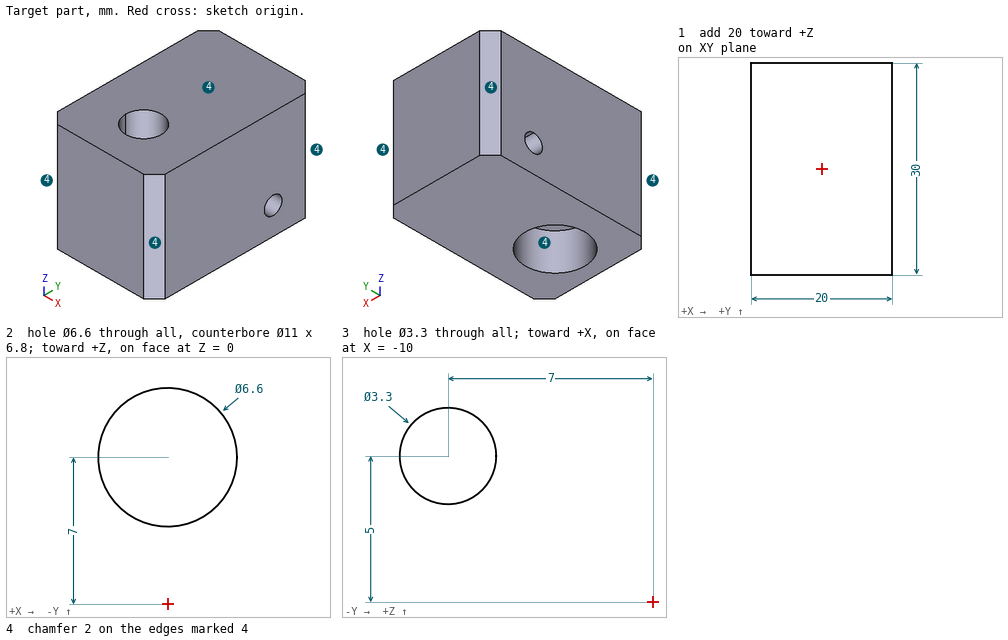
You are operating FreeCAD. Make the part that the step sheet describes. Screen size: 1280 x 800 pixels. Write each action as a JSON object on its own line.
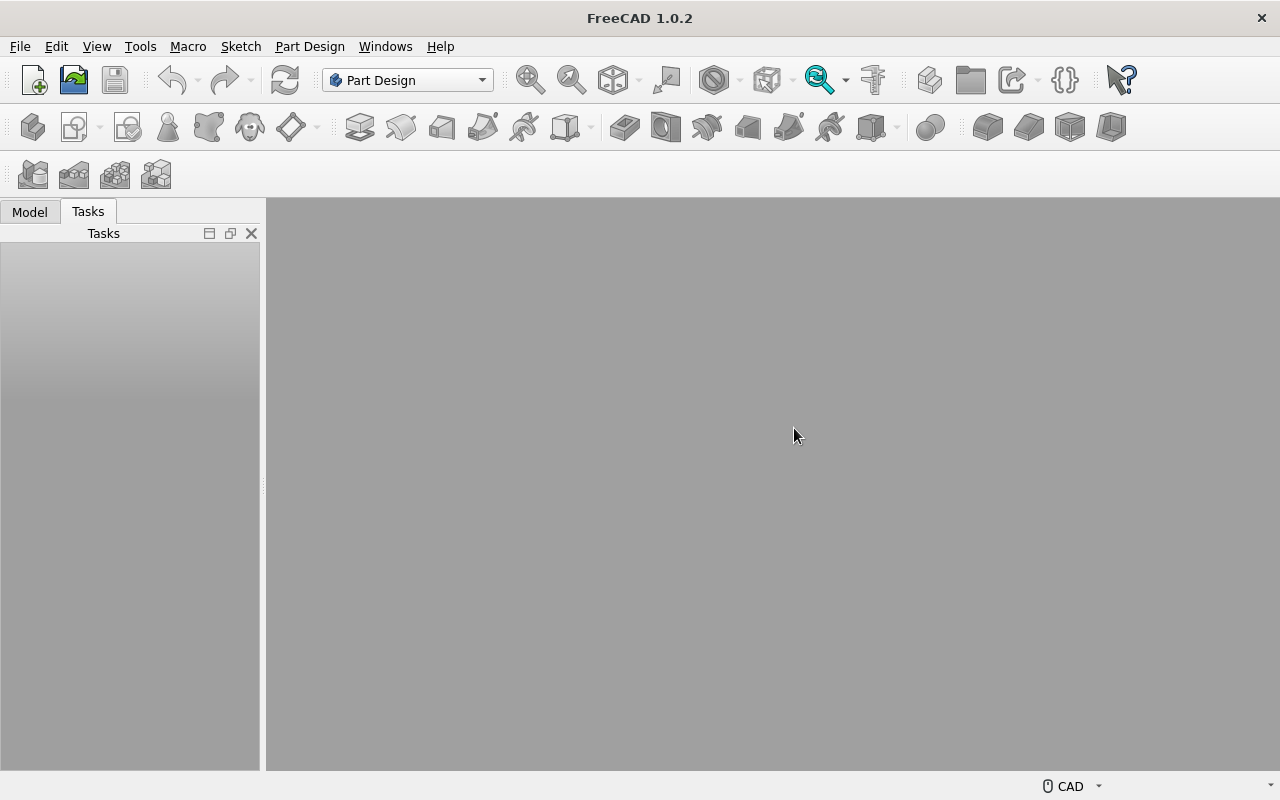
{"action": "key", "text": "ctrl+n"}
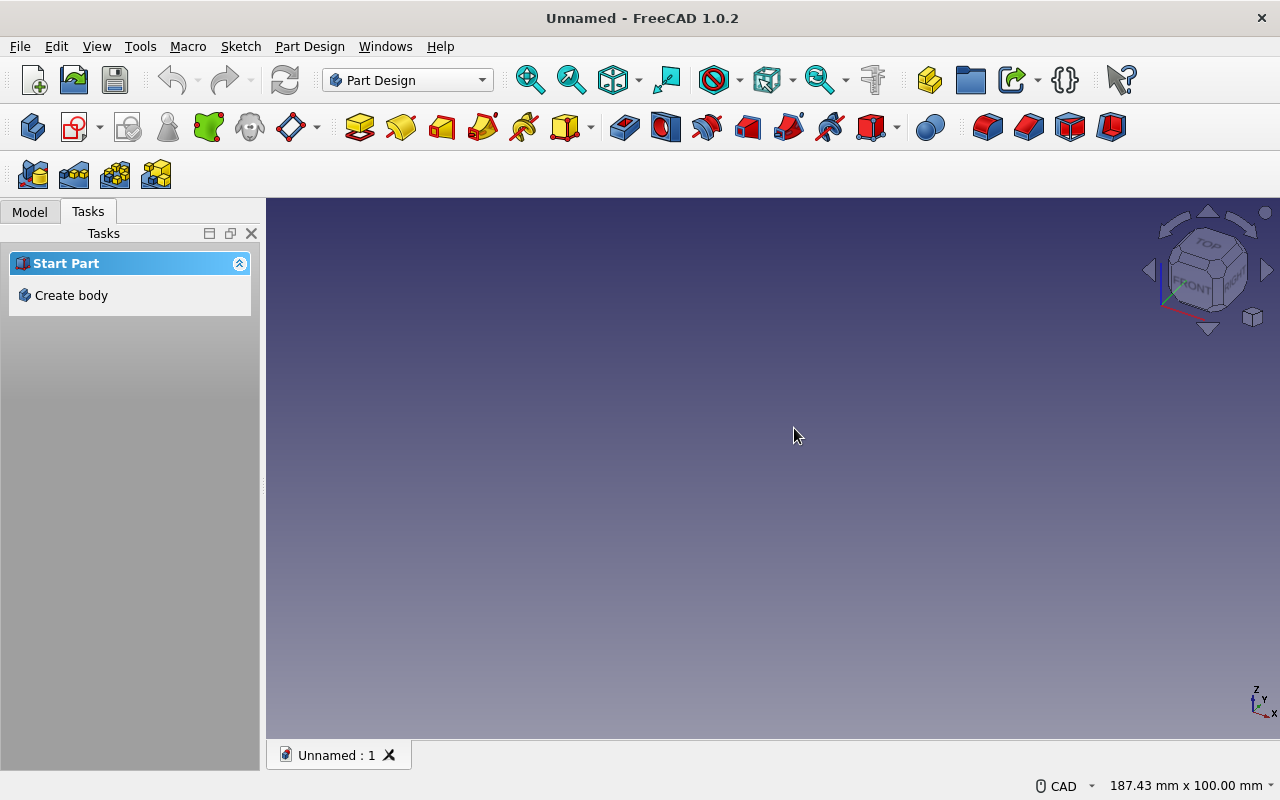
{"action": "left_click", "coordinate": [74, 128]}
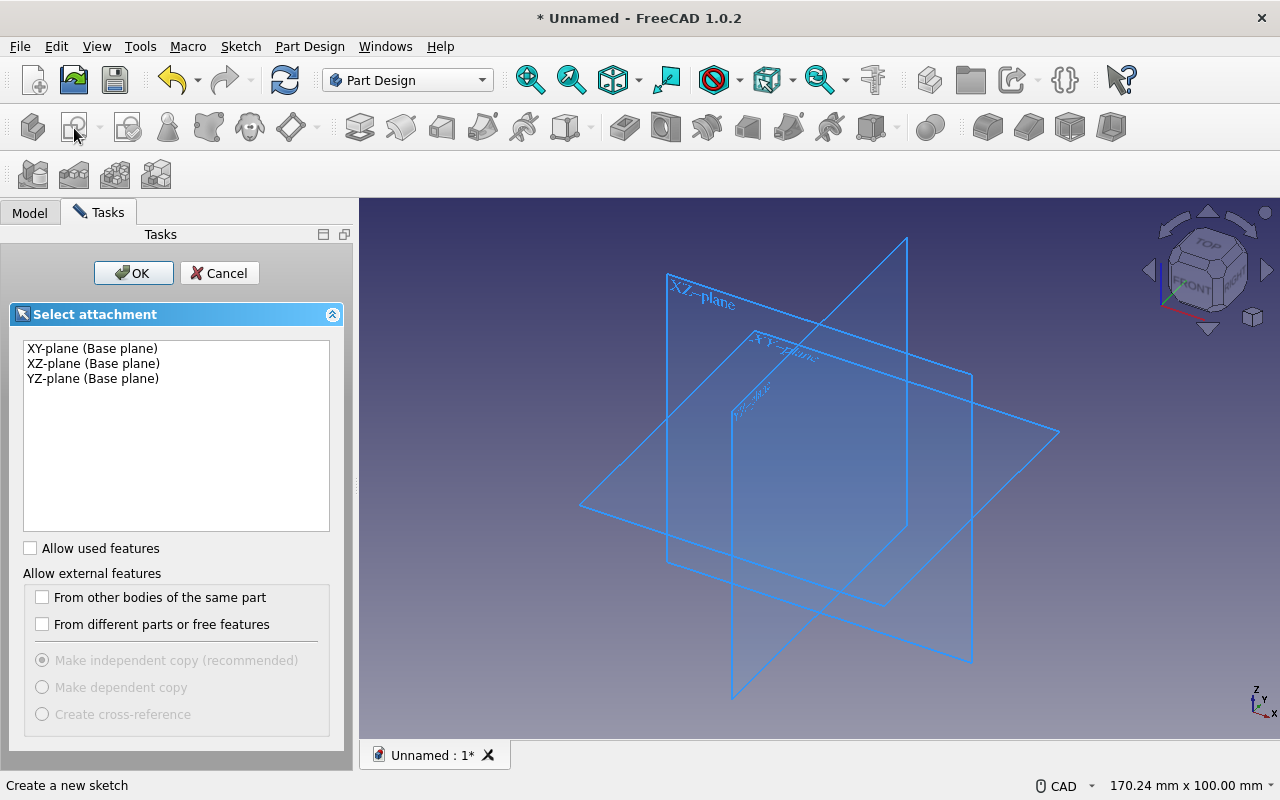
{"action": "left_click", "coordinate": [84, 348]}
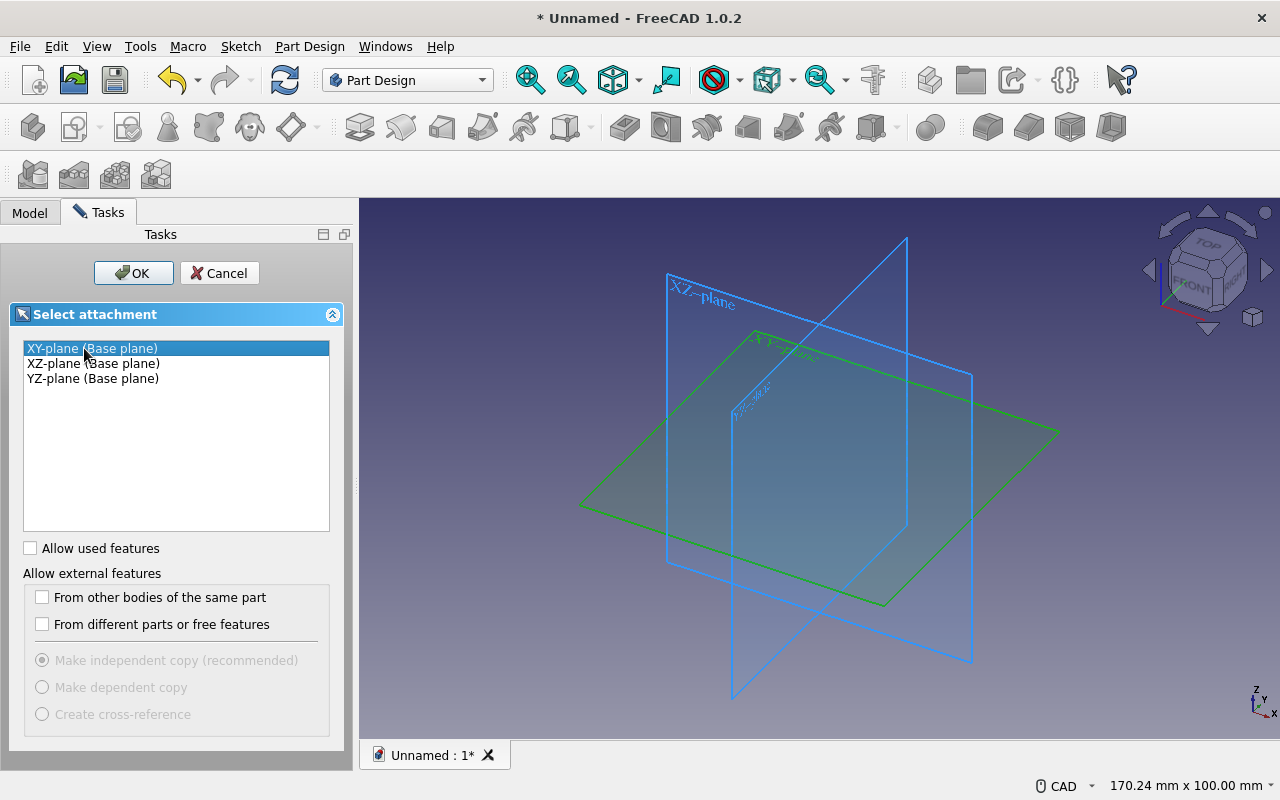
{"action": "left_click", "coordinate": [134, 273]}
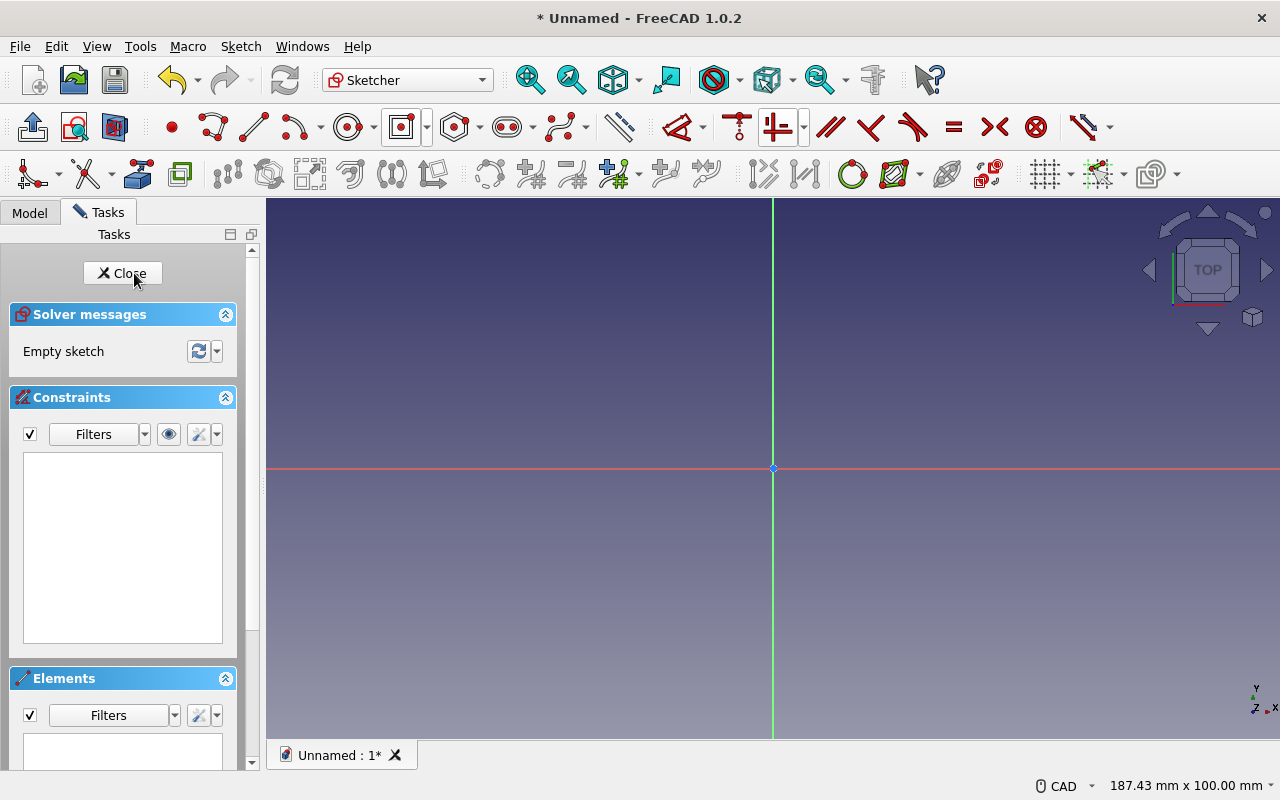
{"action": "scroll", "coordinate": [829, 469], "scroll_direction": "up", "scroll_amount": 4}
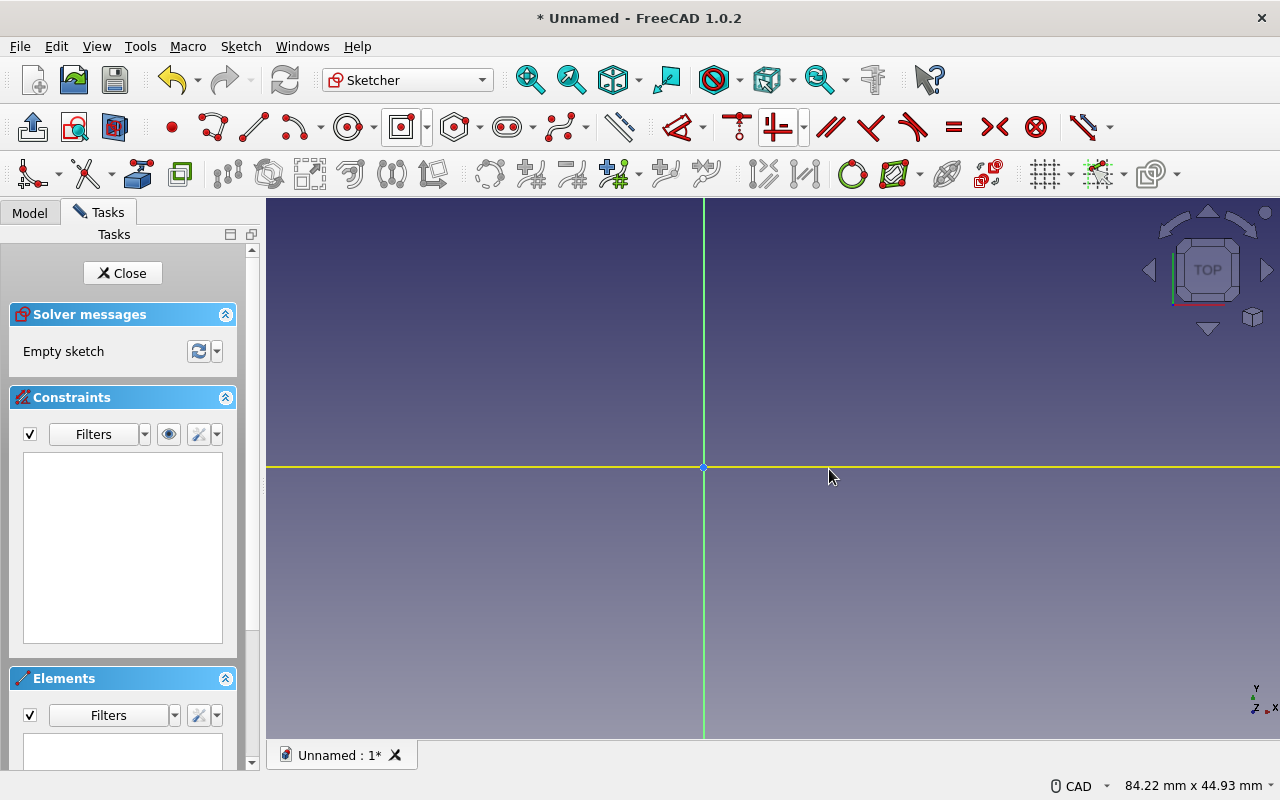
{"action": "key", "text": "g v"}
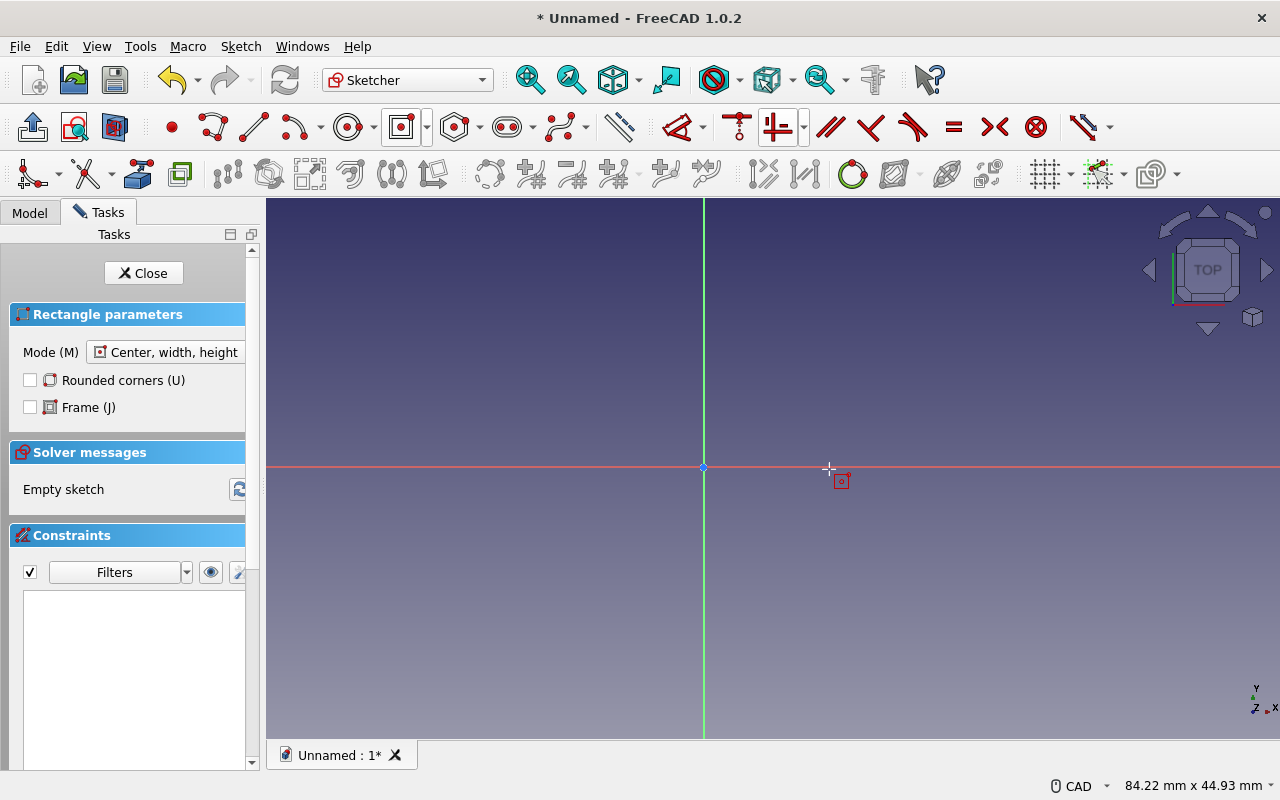
{"action": "left_click", "coordinate": [704, 467]}
{"action": "left_click", "coordinate": [824, 287]}
{"action": "key", "text": "Escape"}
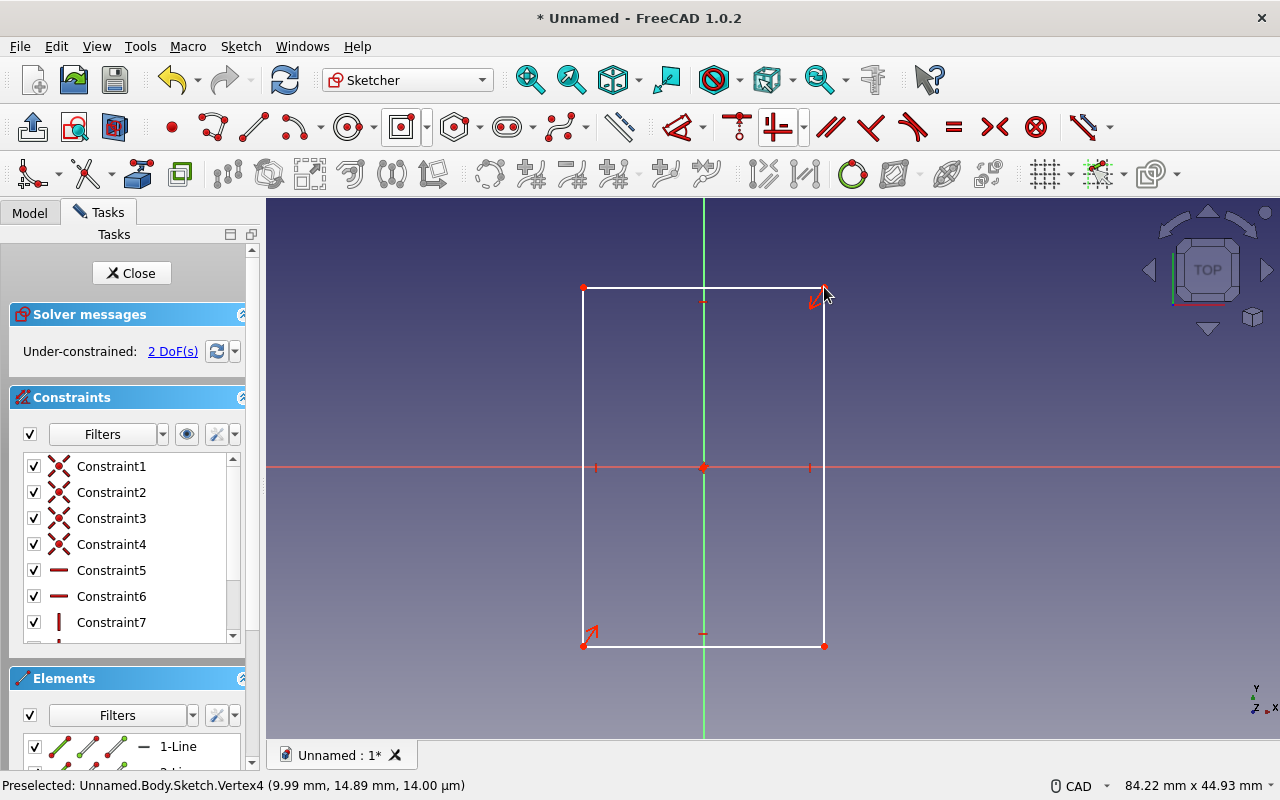
{"action": "left_click", "coordinate": [656, 647]}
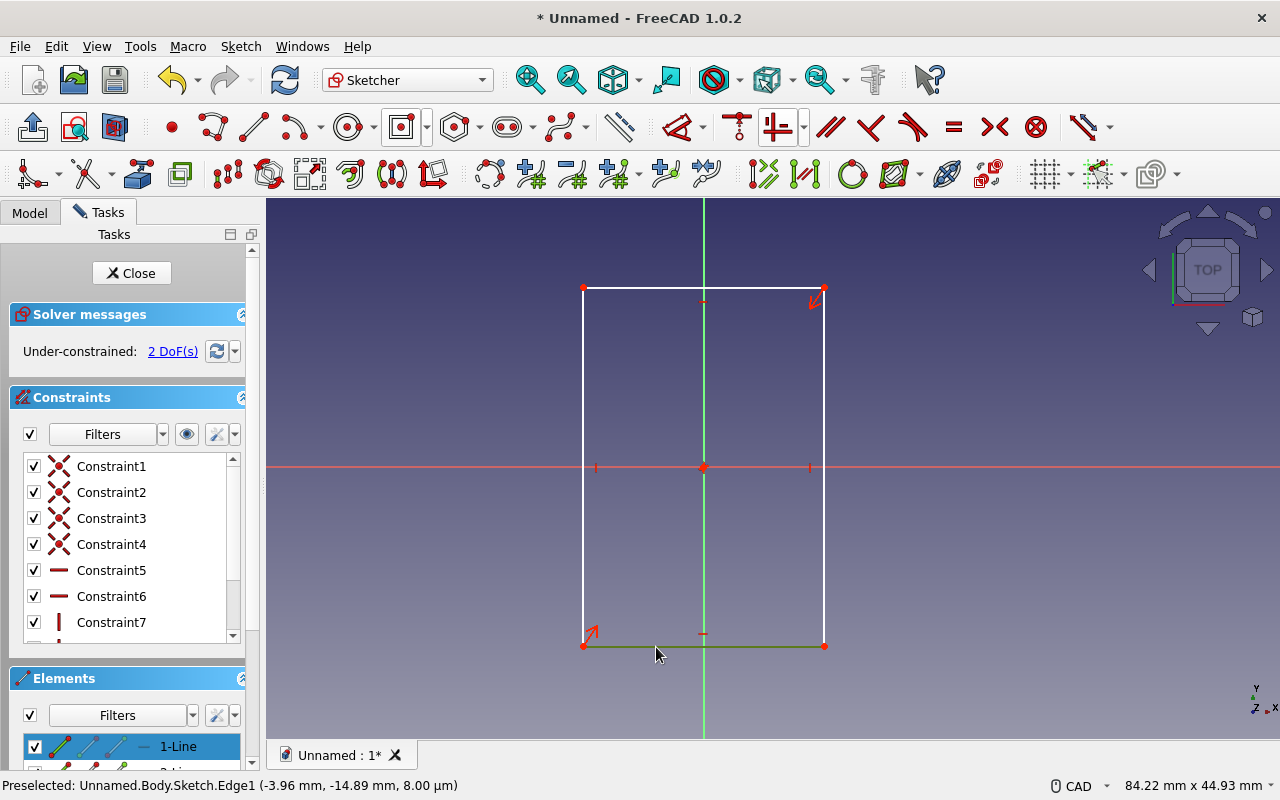
{"action": "key", "text": "l"}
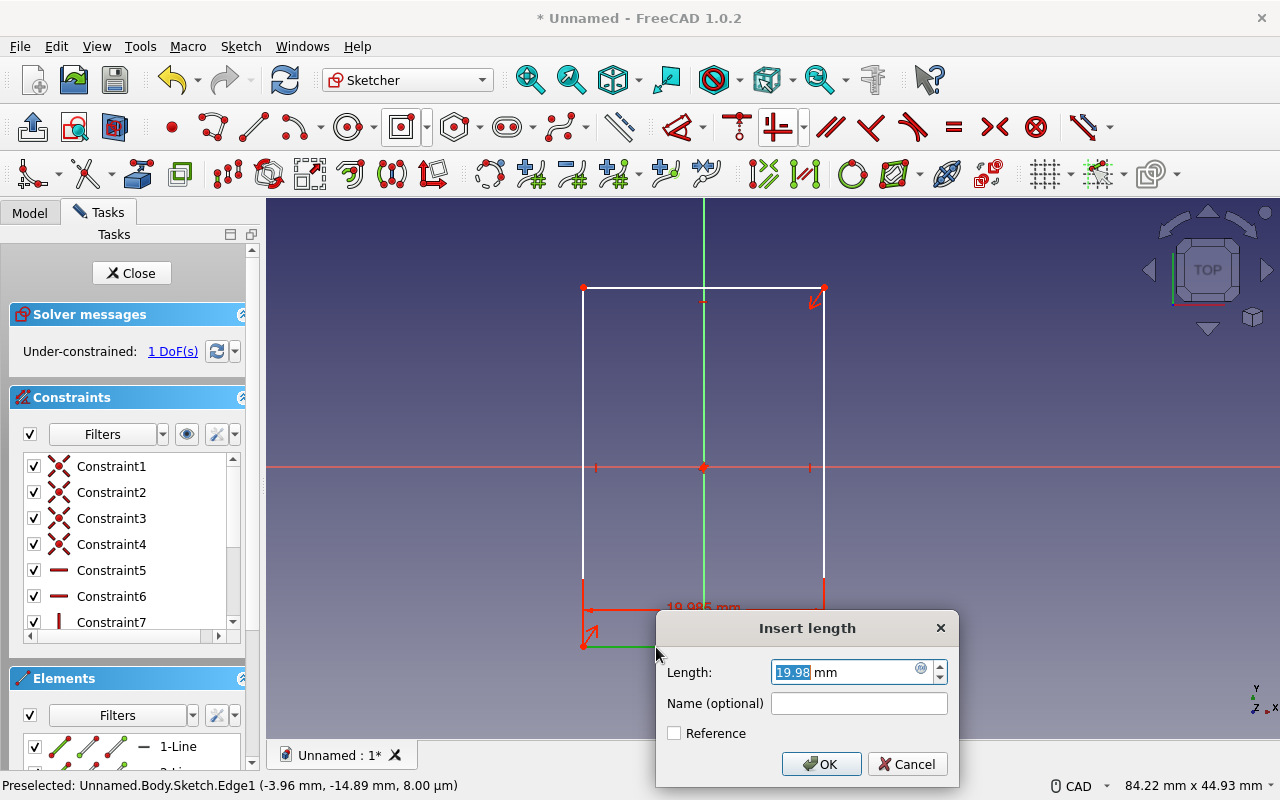
{"action": "type", "text": "20"}
{"action": "key", "text": "Return"}